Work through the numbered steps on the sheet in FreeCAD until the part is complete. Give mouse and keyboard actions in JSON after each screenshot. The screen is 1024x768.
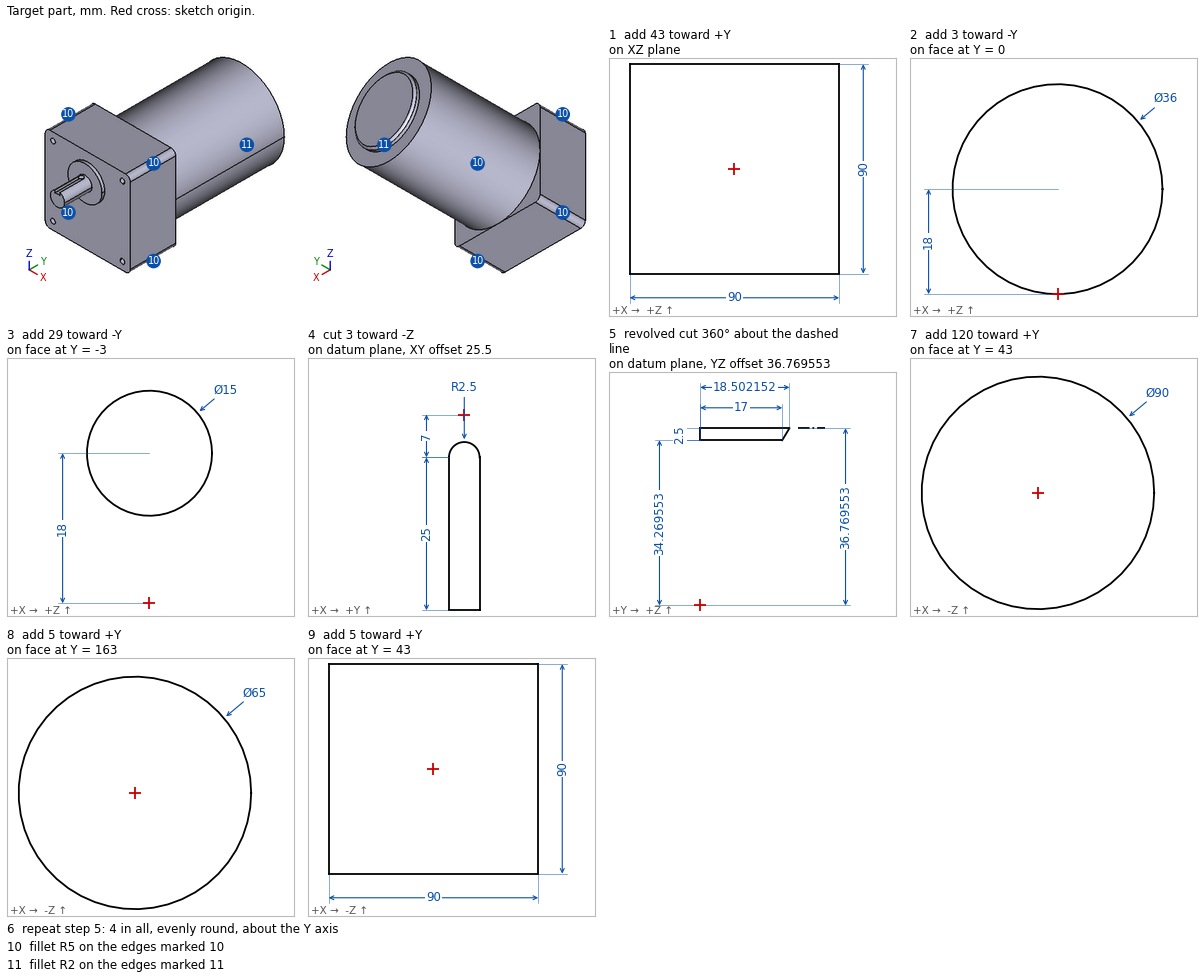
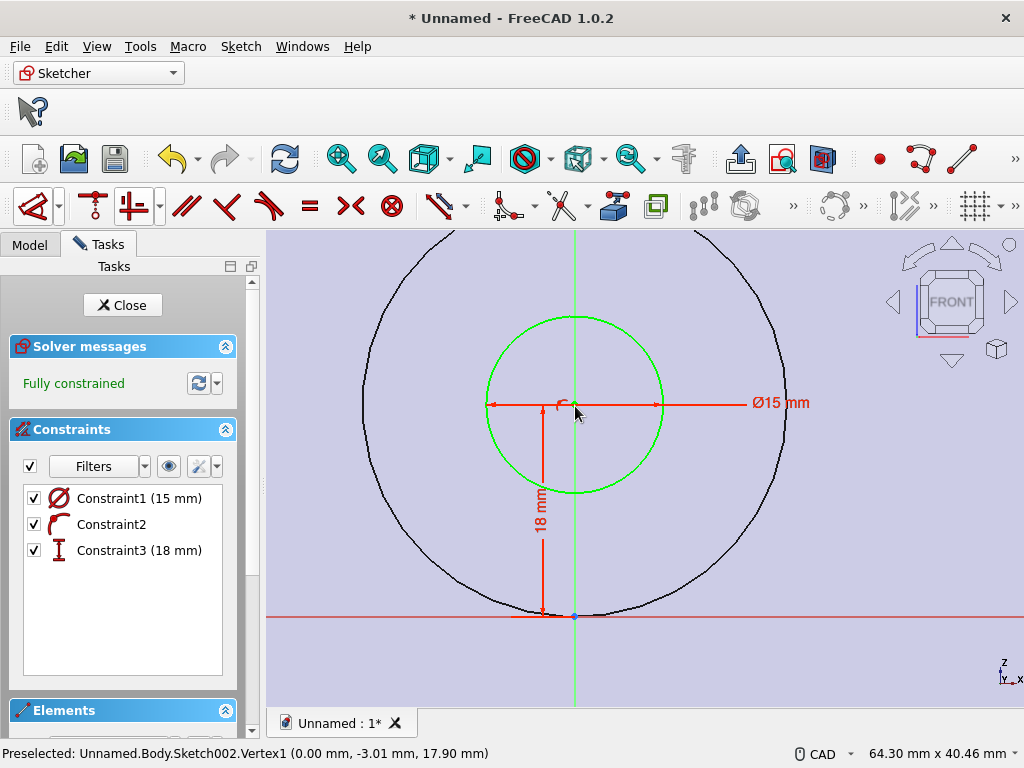
{"action": "left_click", "coordinate": [123, 305]}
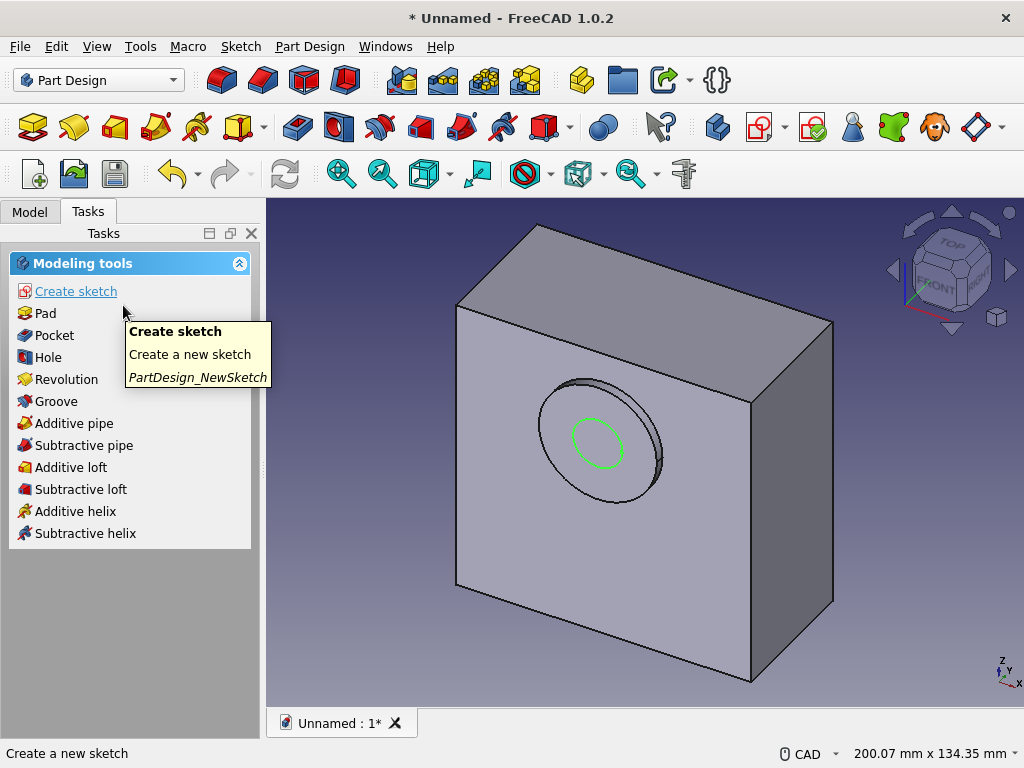
{"action": "left_click", "coordinate": [33, 128]}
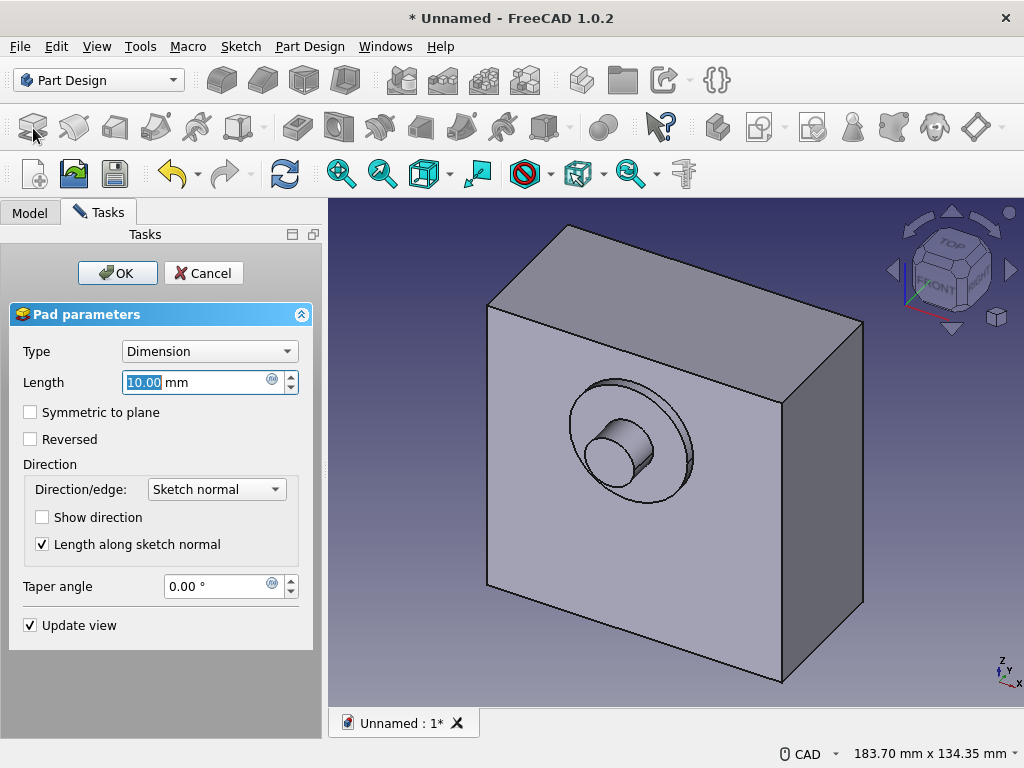
{"action": "type", "text": "29"}
{"action": "key", "text": "Tab"}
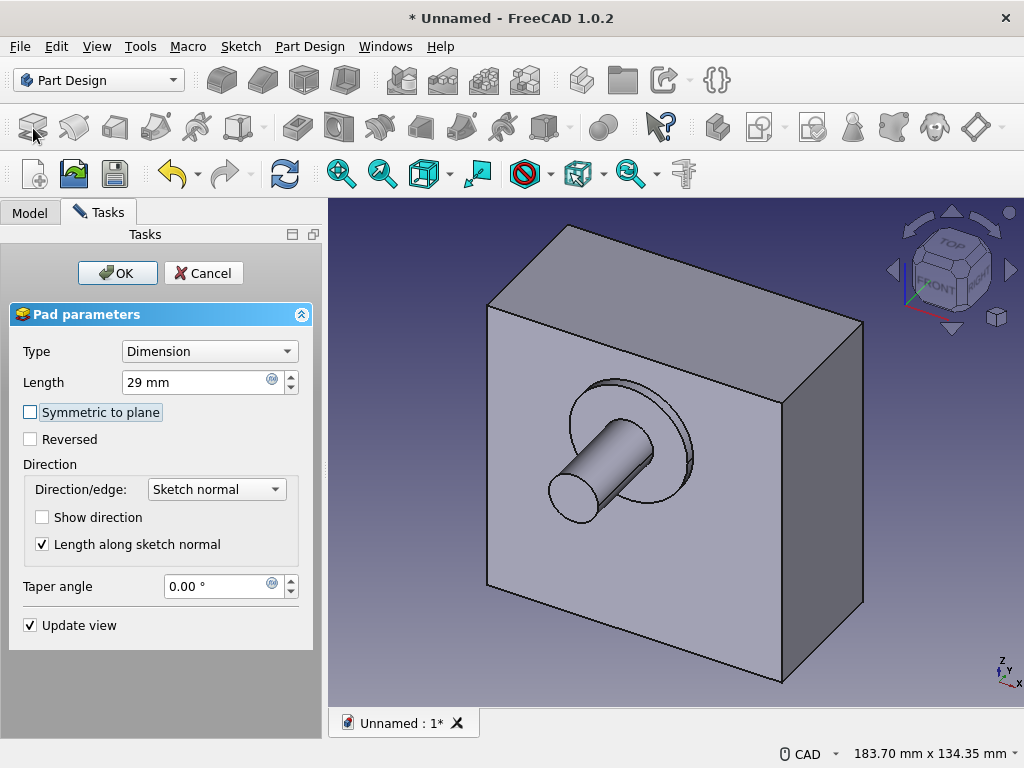
{"action": "left_click", "coordinate": [118, 273]}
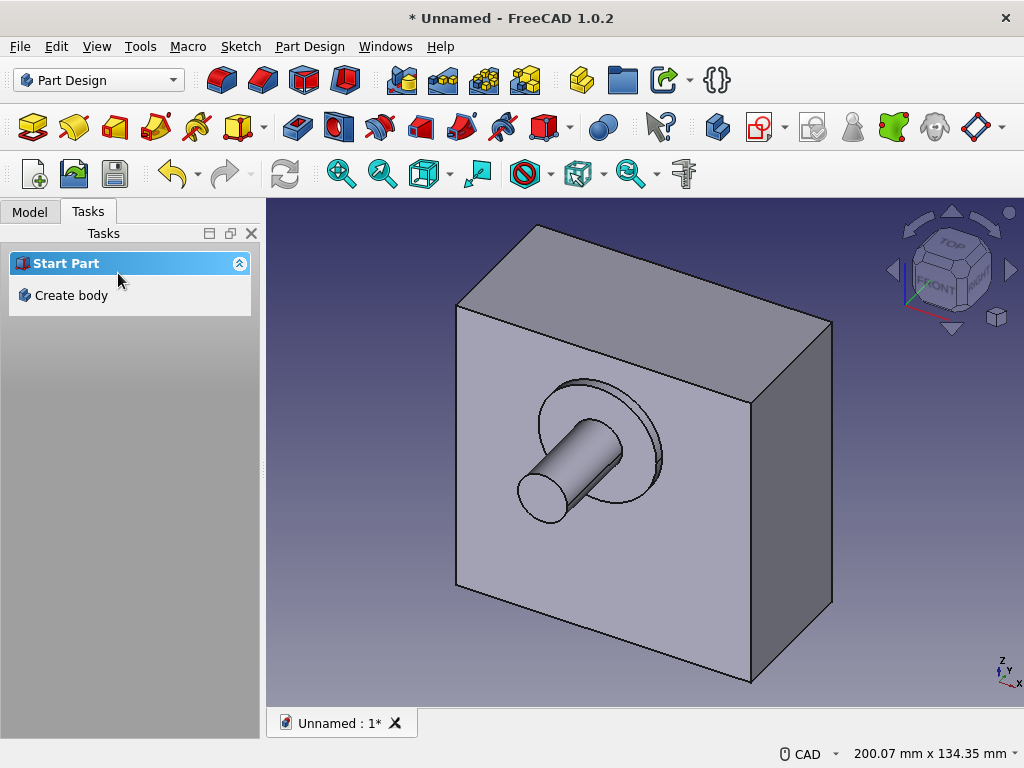
{"action": "left_click", "coordinate": [342, 174]}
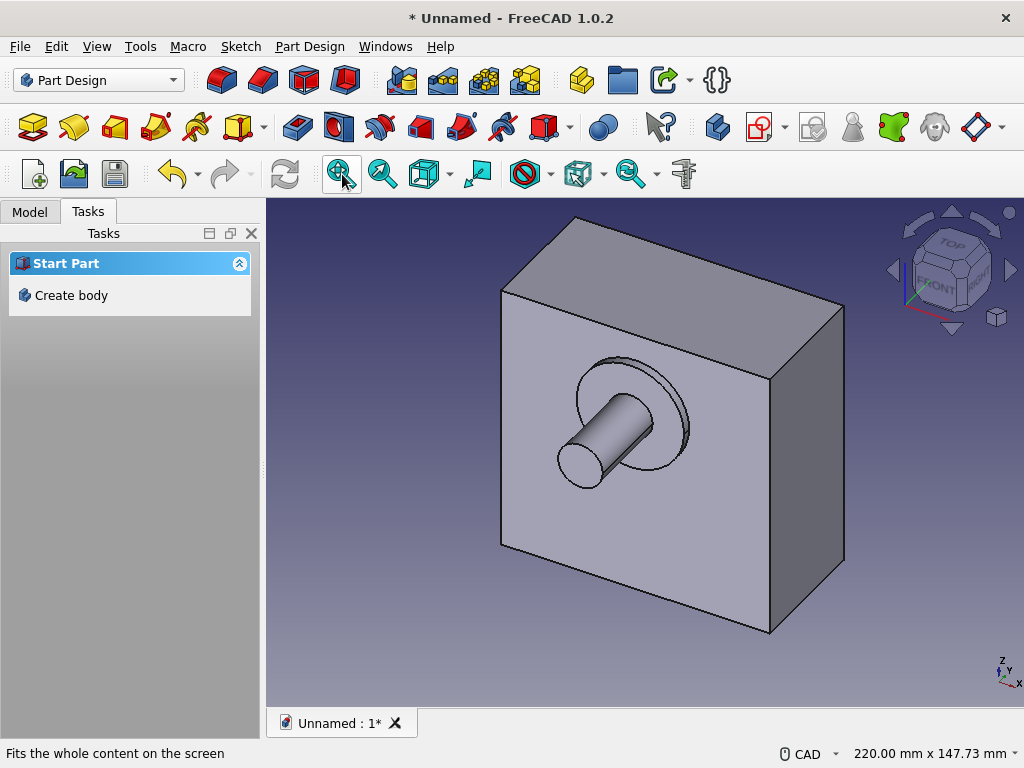
{"action": "left_click", "coordinate": [30, 212]}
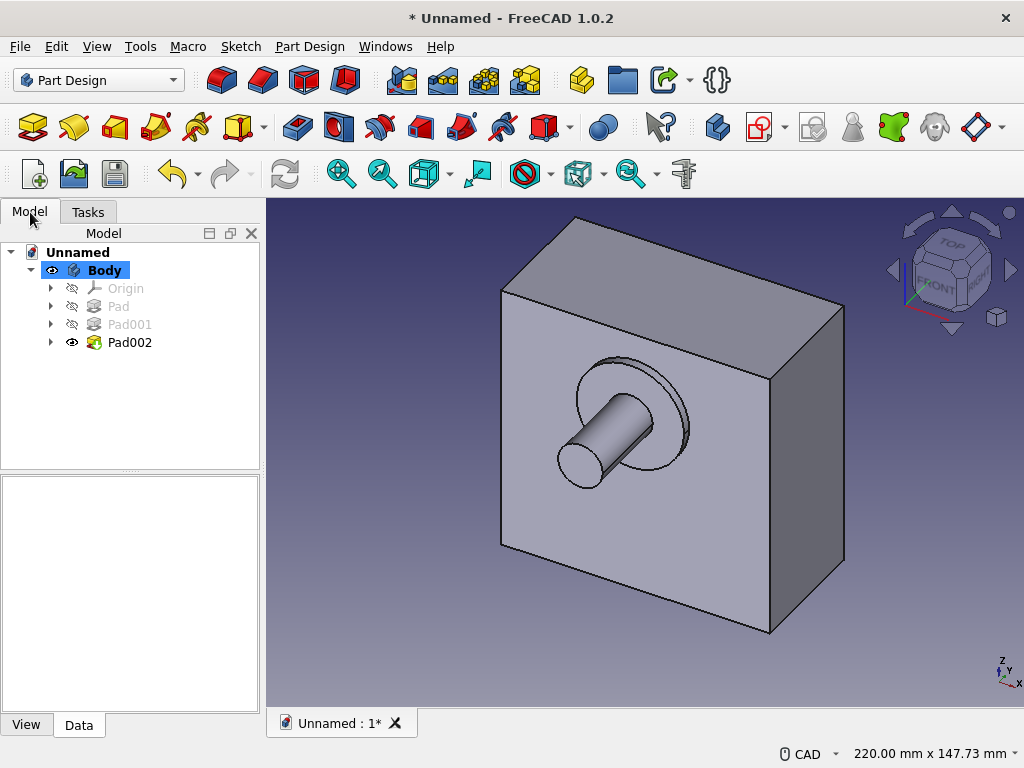
{"action": "left_click", "coordinate": [51, 288]}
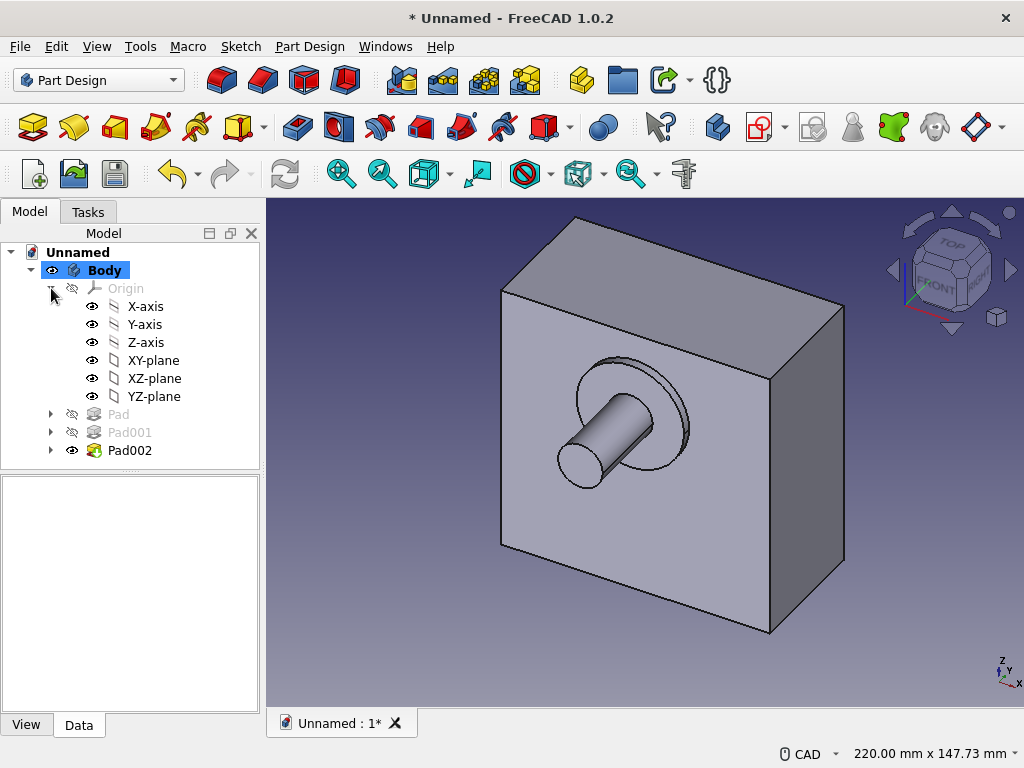
{"action": "left_click", "coordinate": [137, 360]}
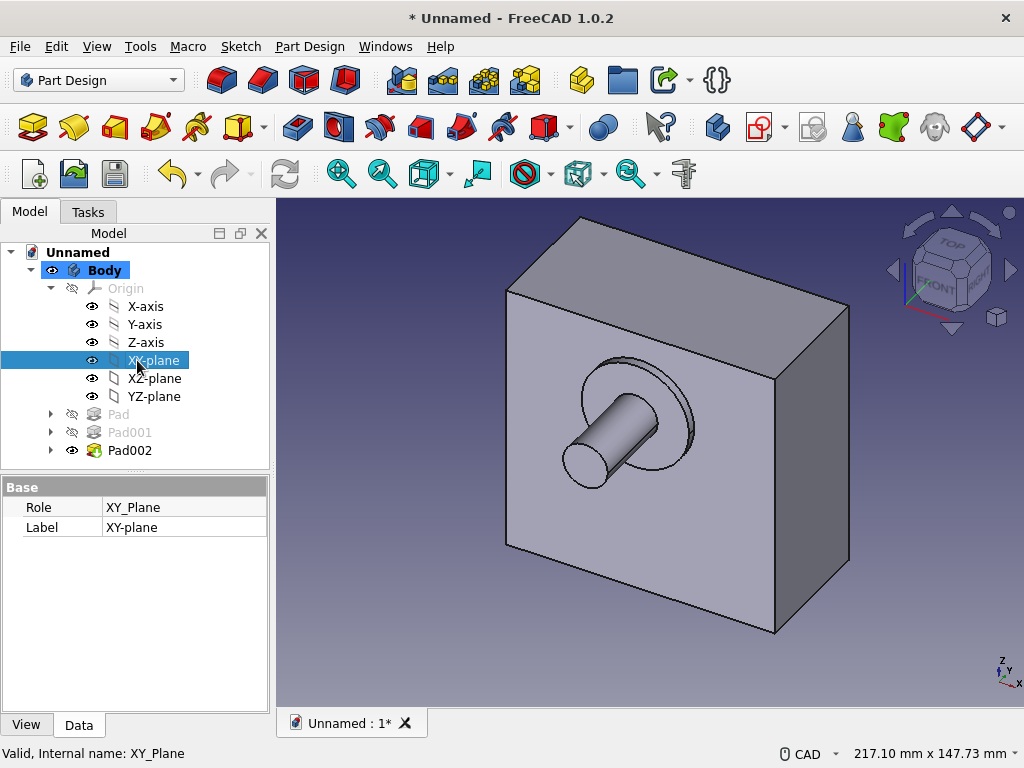
{"action": "left_click", "coordinate": [976, 128]}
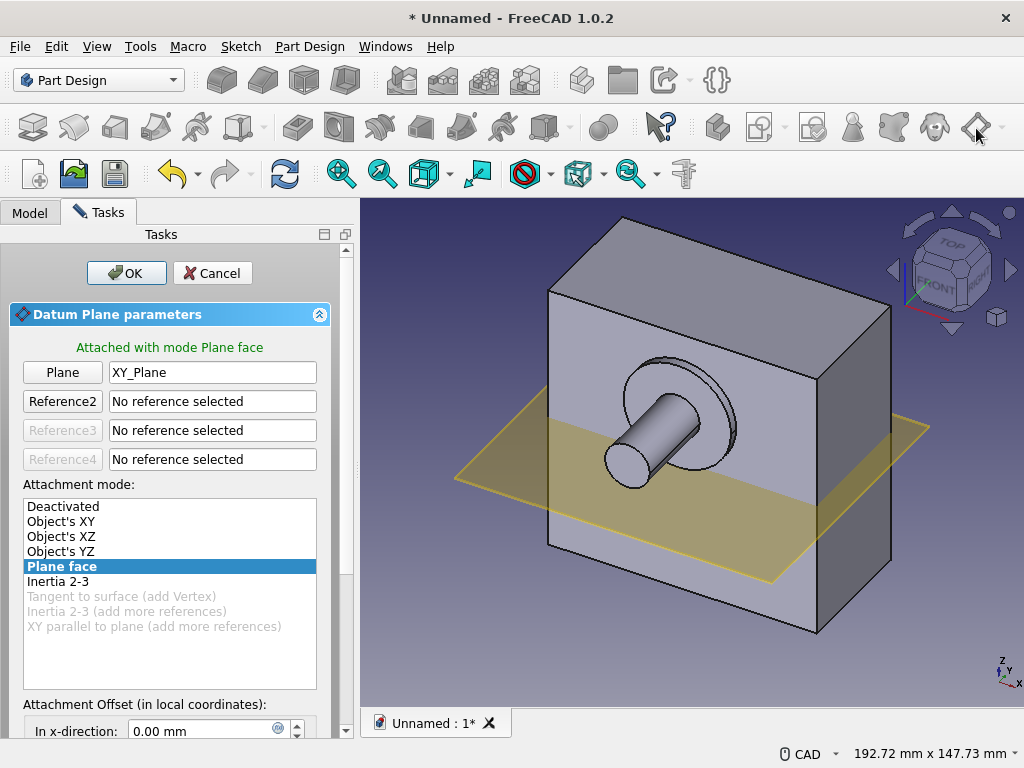
{"action": "scroll", "coordinate": [346, 491], "scroll_direction": "down", "scroll_amount": 3}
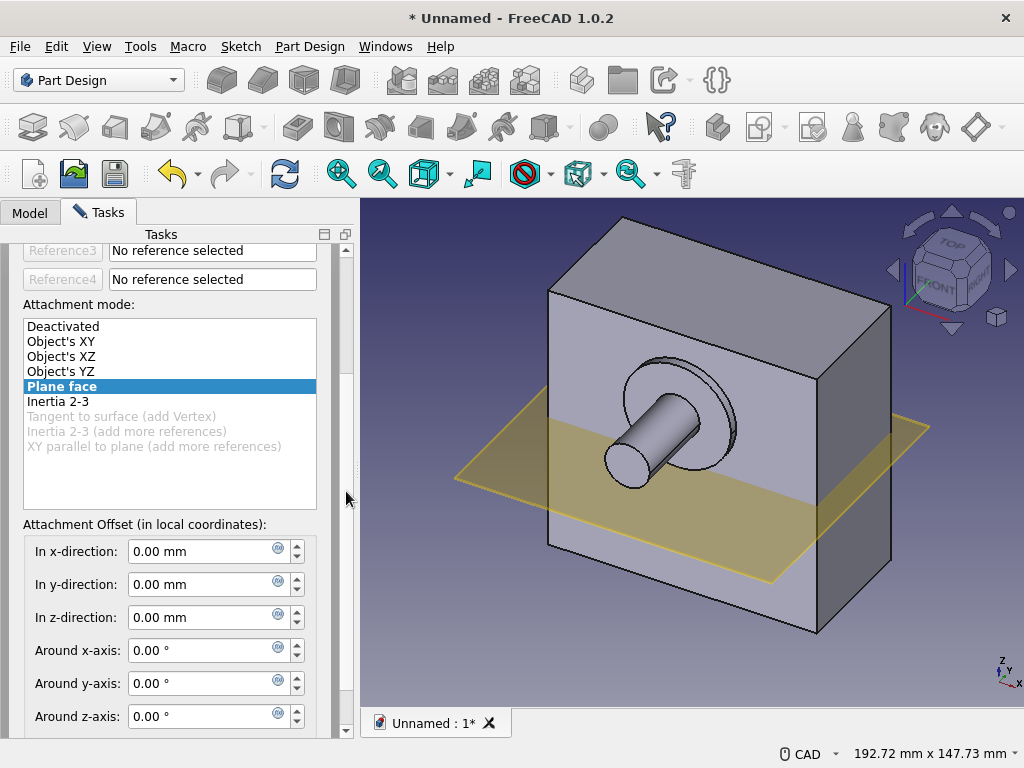
{"action": "triple_click", "coordinate": [210, 618]}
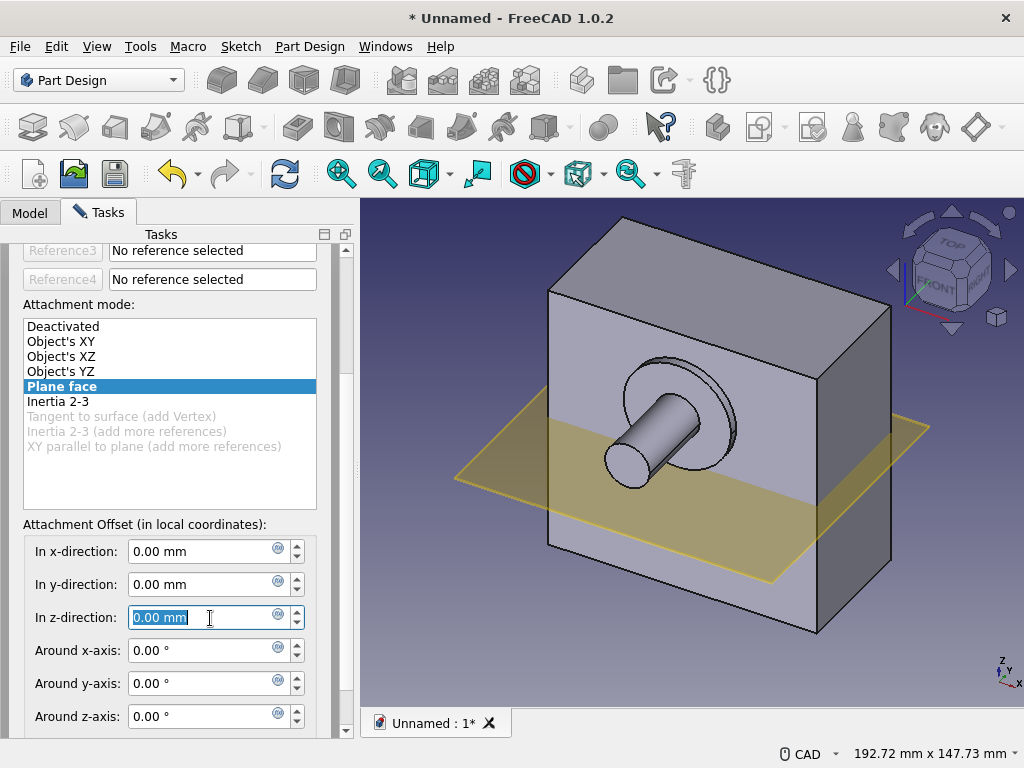
{"action": "type", "text": "25.5"}
{"action": "key", "text": "Tab"}